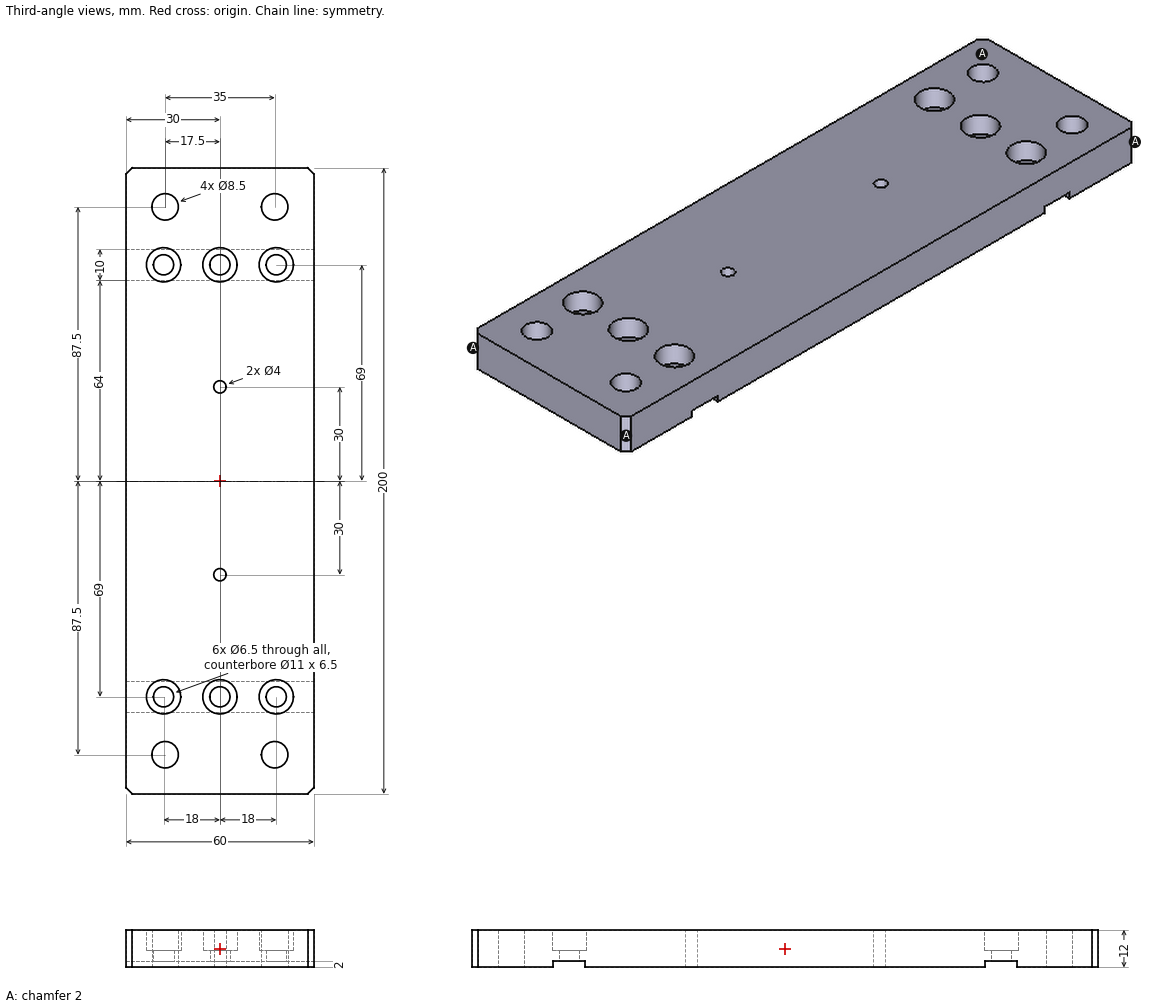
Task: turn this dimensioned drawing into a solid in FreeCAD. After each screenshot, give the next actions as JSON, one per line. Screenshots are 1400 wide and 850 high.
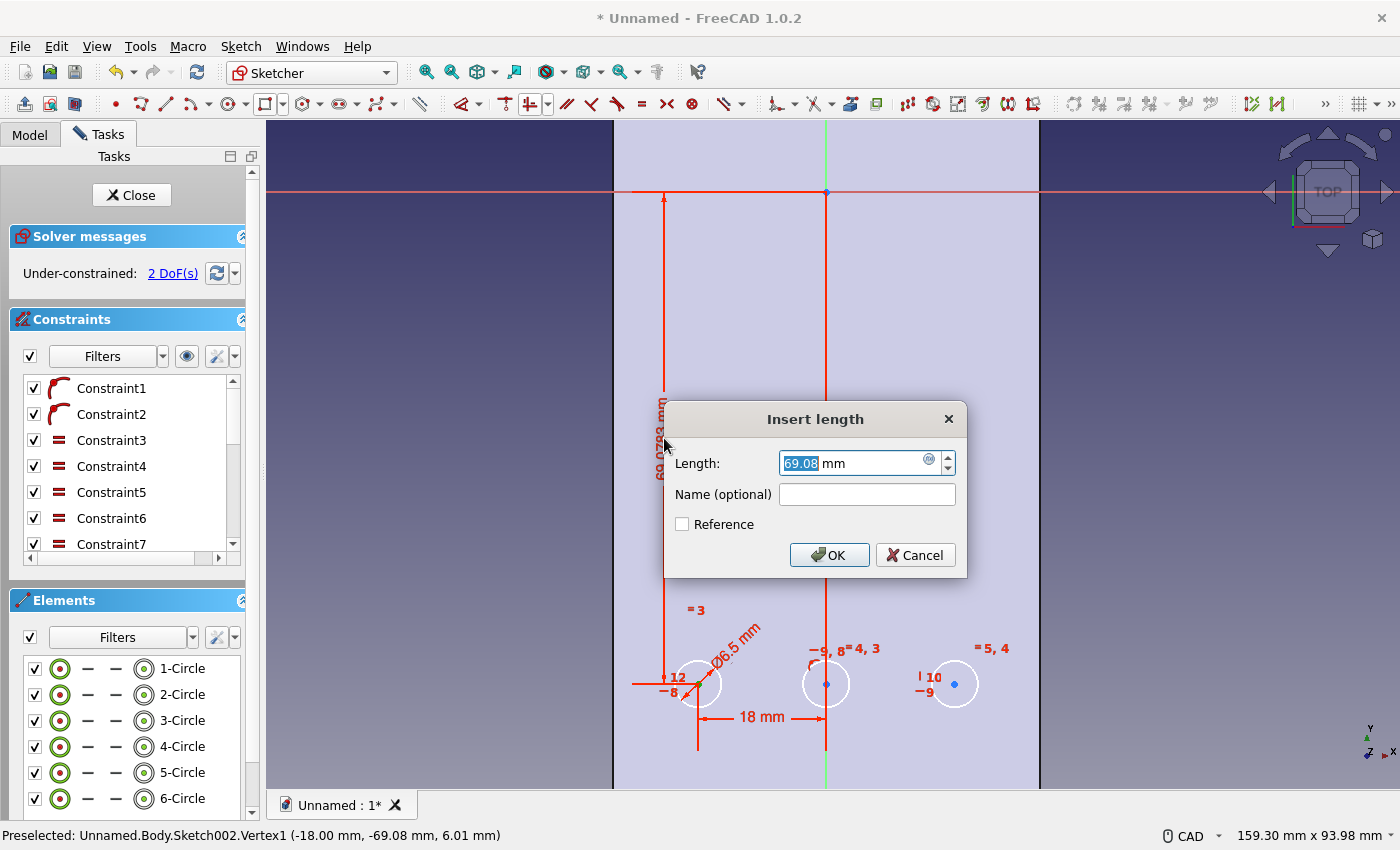
{"action": "type", "text": "69"}
{"action": "key", "text": "Return"}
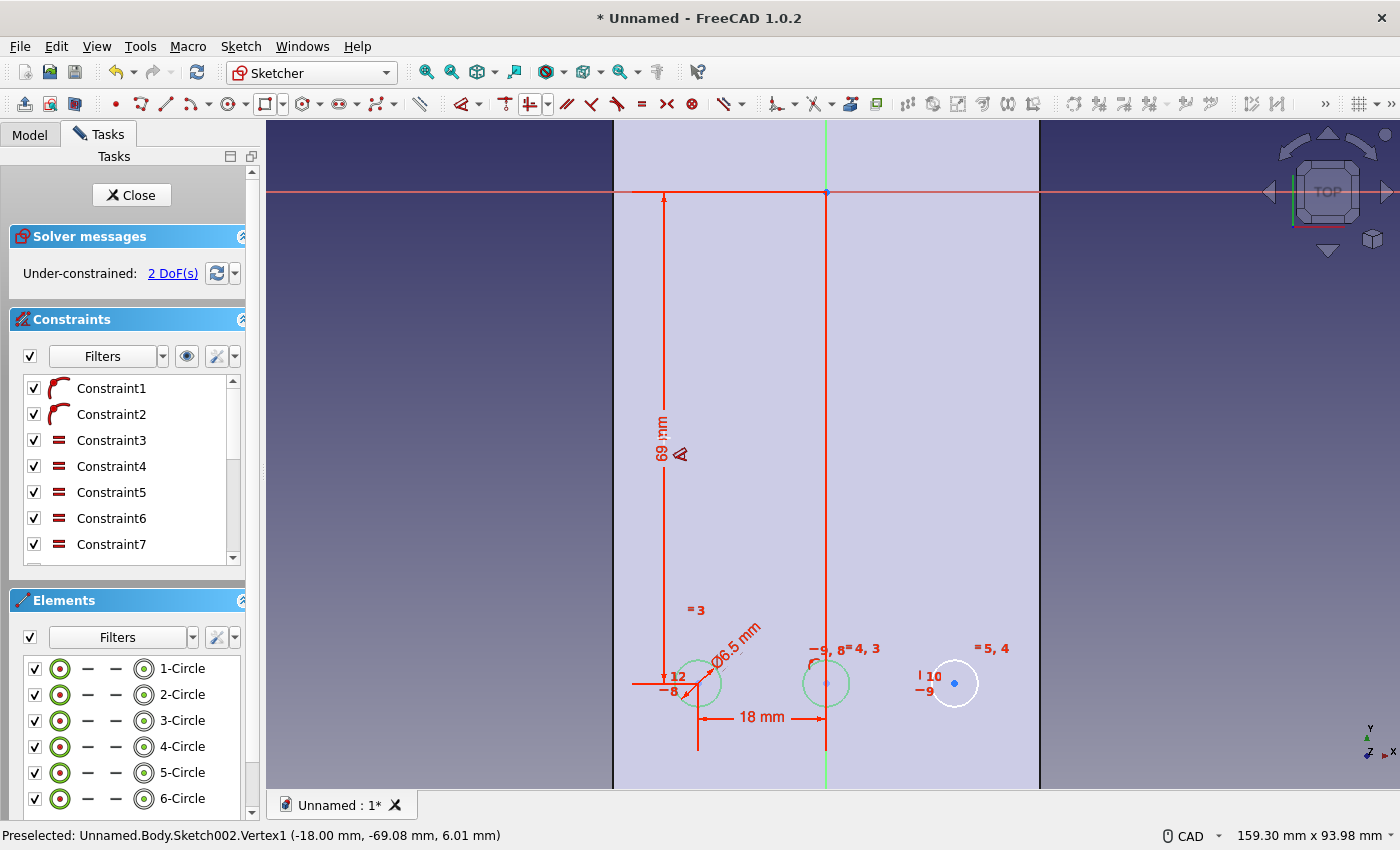
{"action": "left_click", "coordinate": [955, 684]}
{"action": "left_click", "coordinate": [890, 718]}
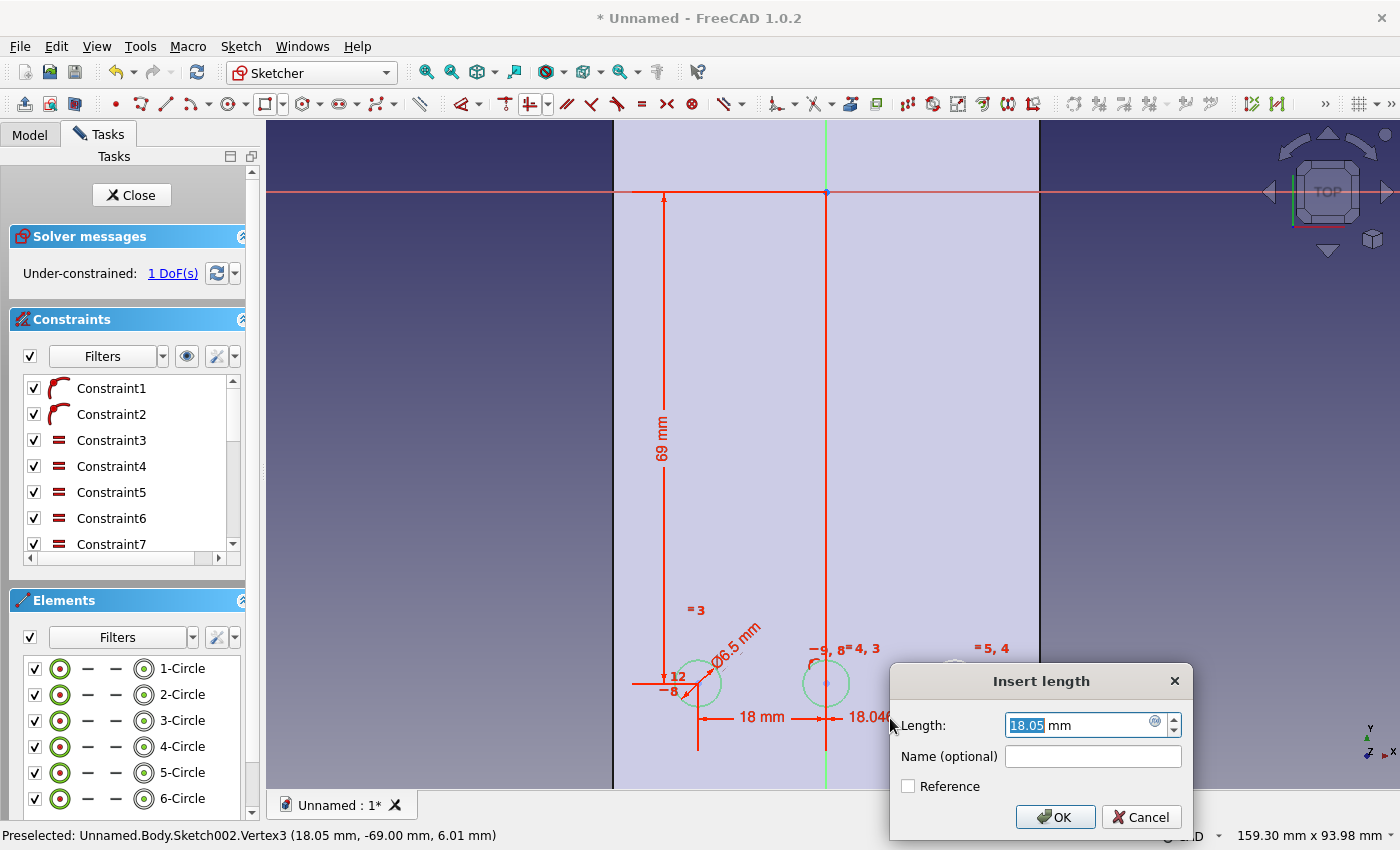
{"action": "type", "text": "18"}
{"action": "key", "text": "Return"}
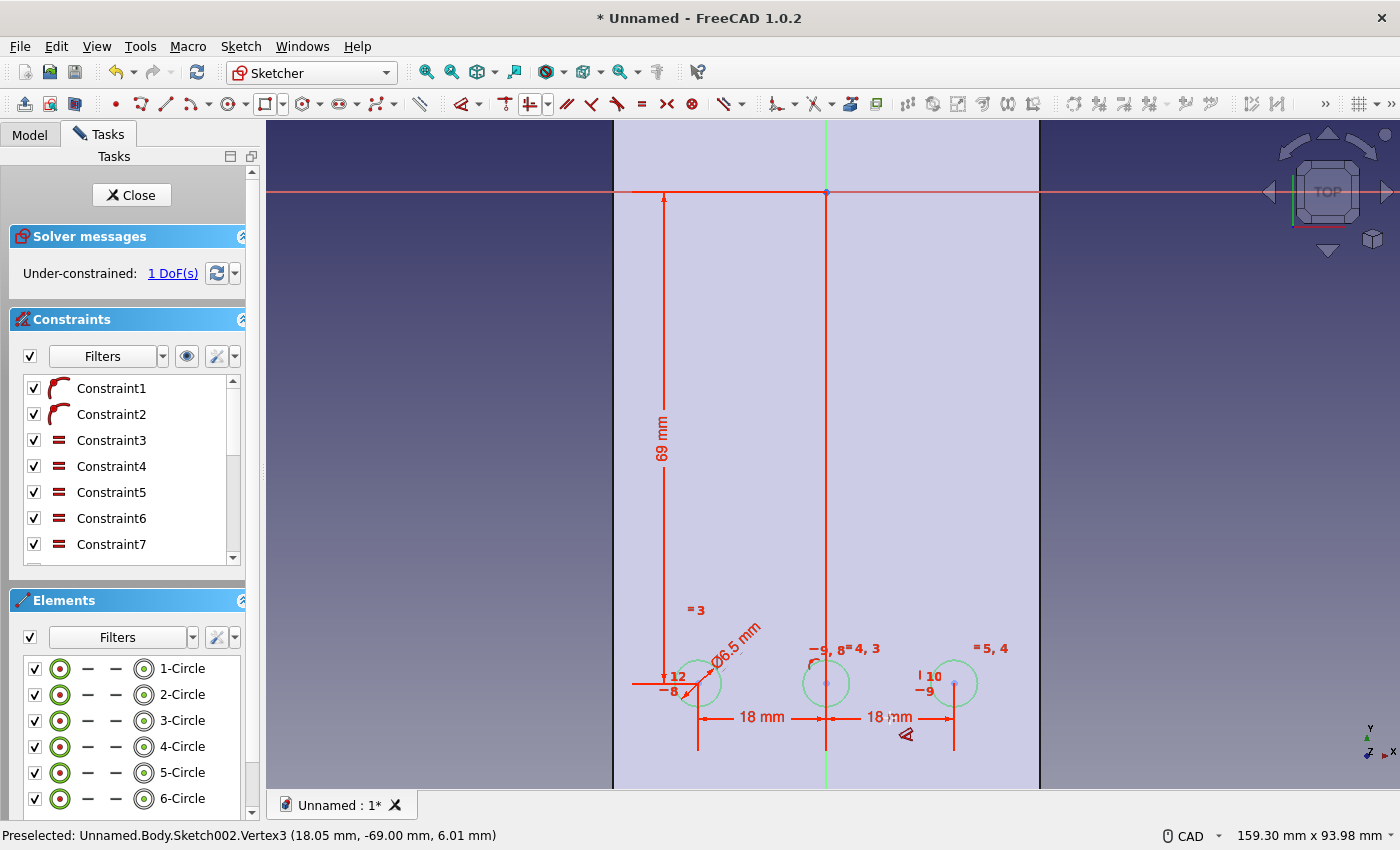
{"action": "scroll", "coordinate": [714, 668], "scroll_direction": "down", "scroll_amount": 4}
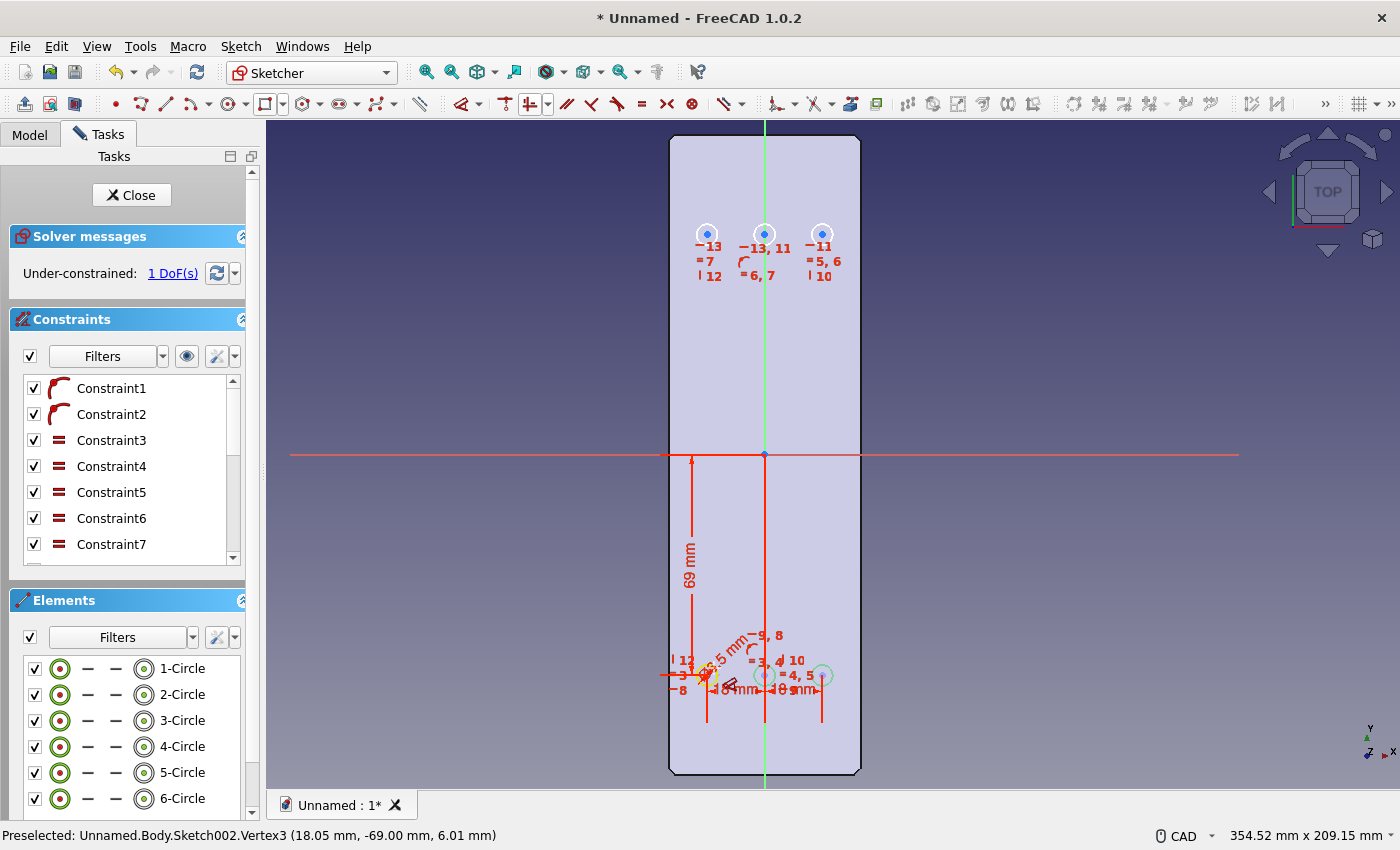
{"action": "left_click", "coordinate": [822, 235]}
{"action": "left_click", "coordinate": [856, 345]}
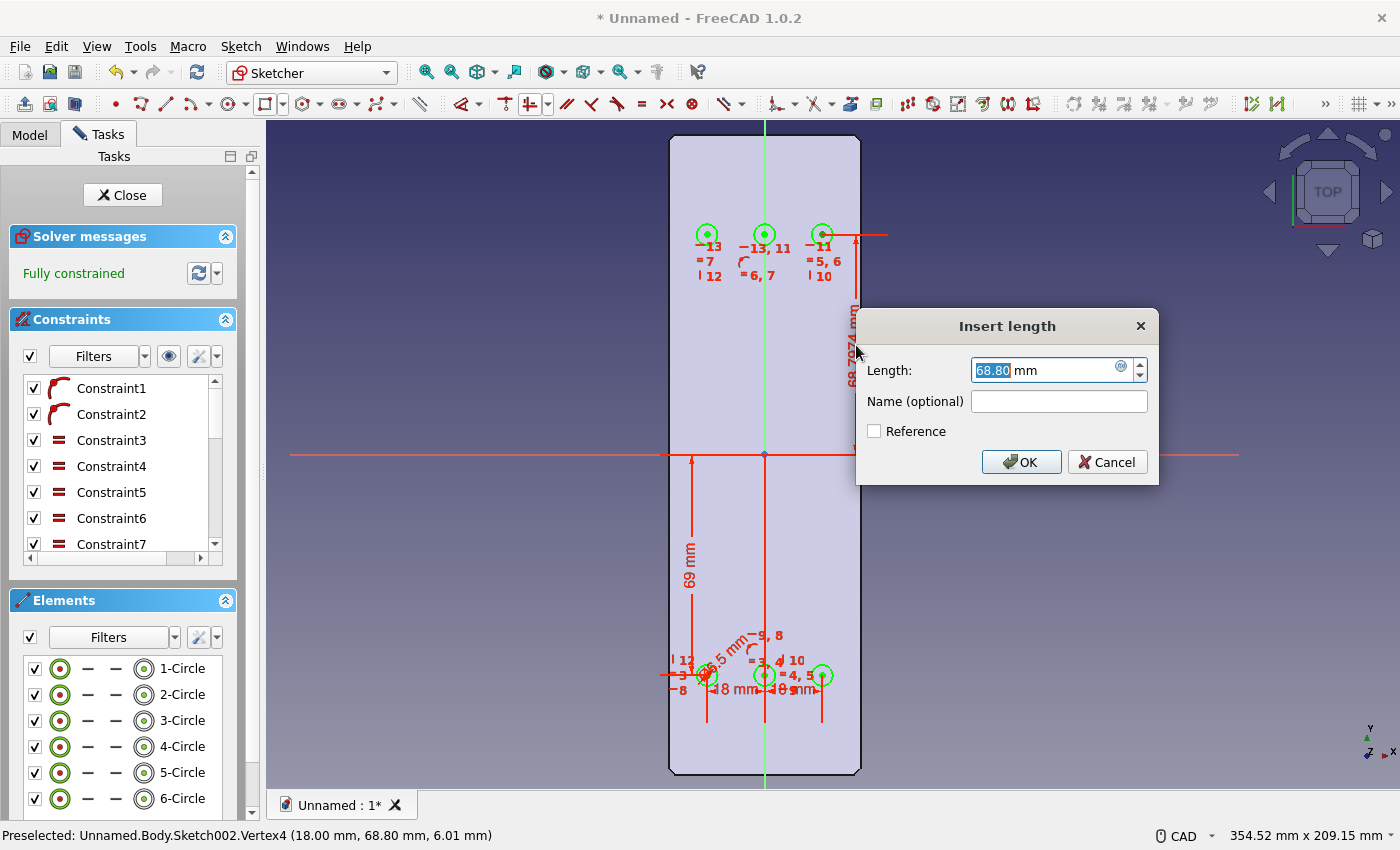
{"action": "type", "text": "69"}
{"action": "key", "text": "Return"}
{"action": "key", "text": "Escape"}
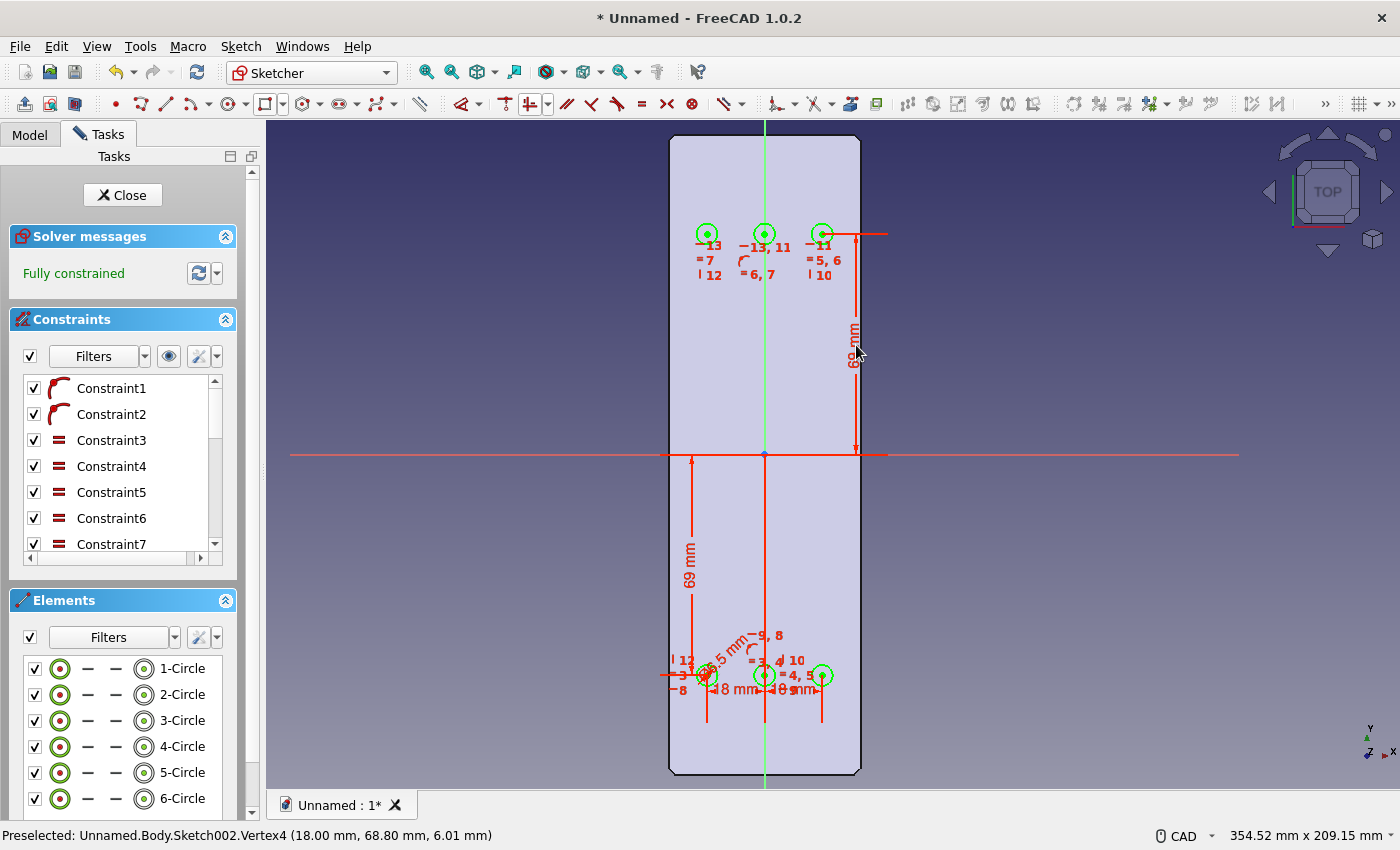
{"action": "left_click", "coordinate": [123, 195]}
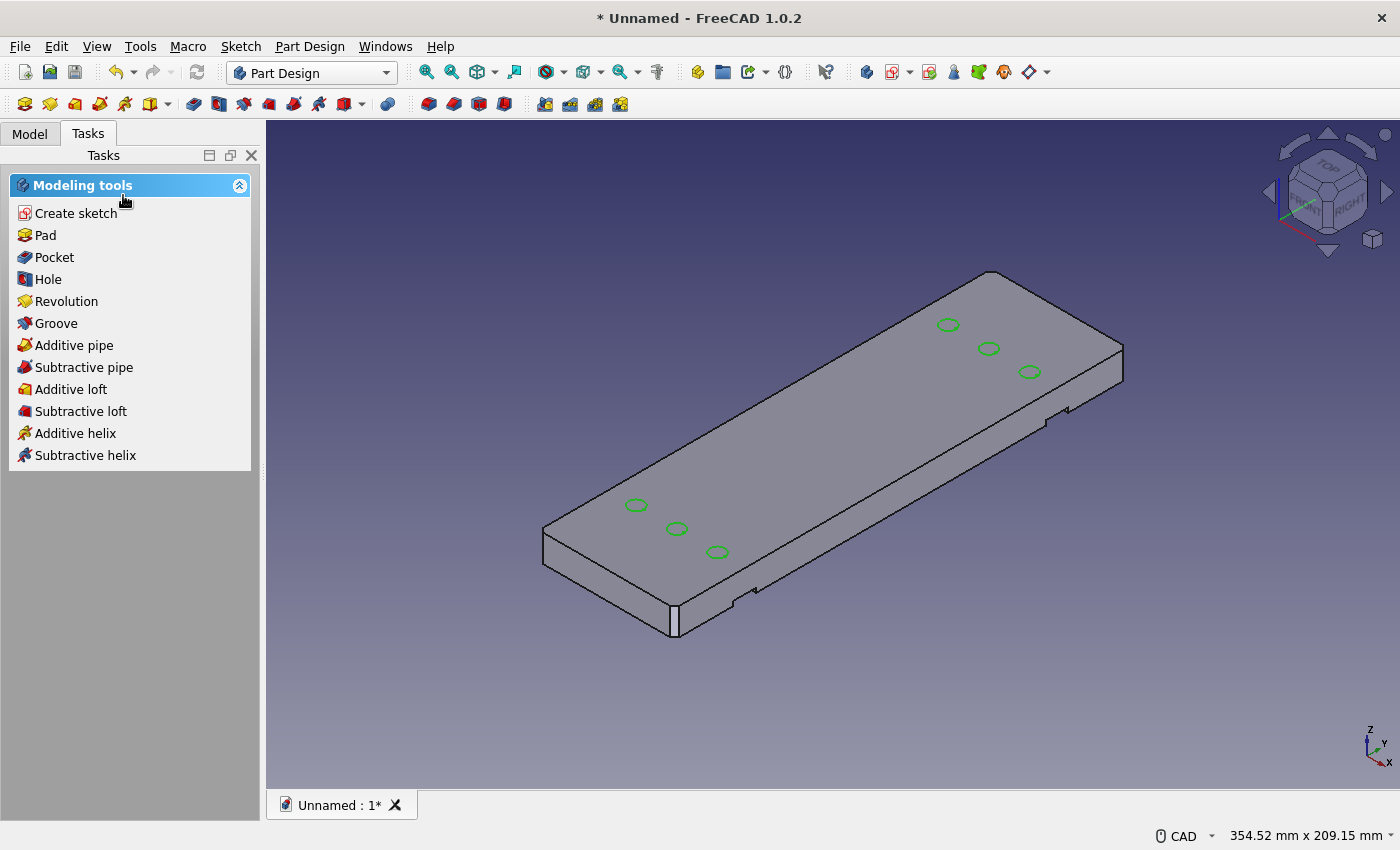
{"action": "left_click", "coordinate": [219, 104]}